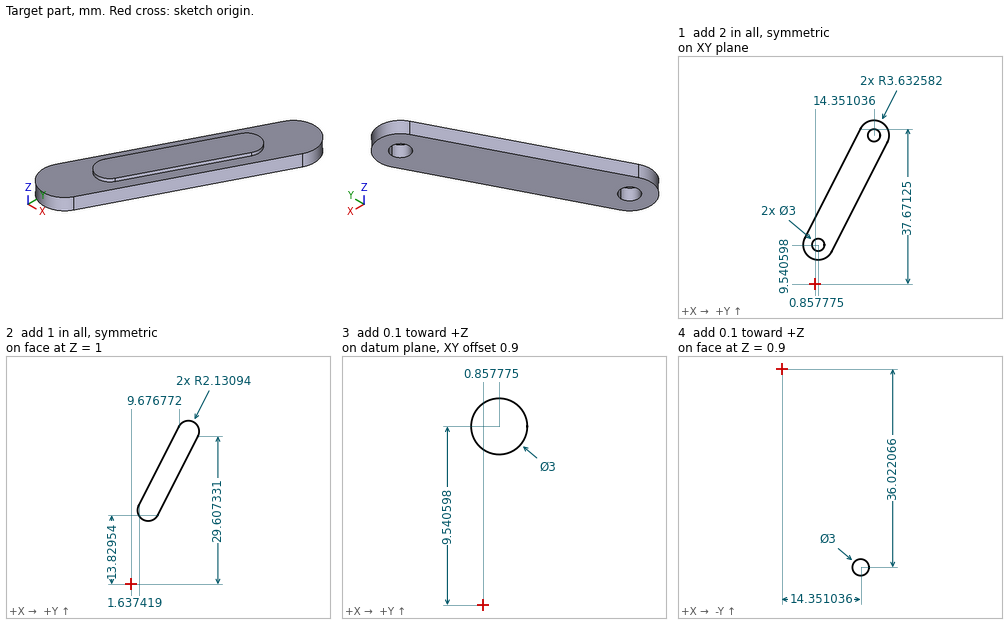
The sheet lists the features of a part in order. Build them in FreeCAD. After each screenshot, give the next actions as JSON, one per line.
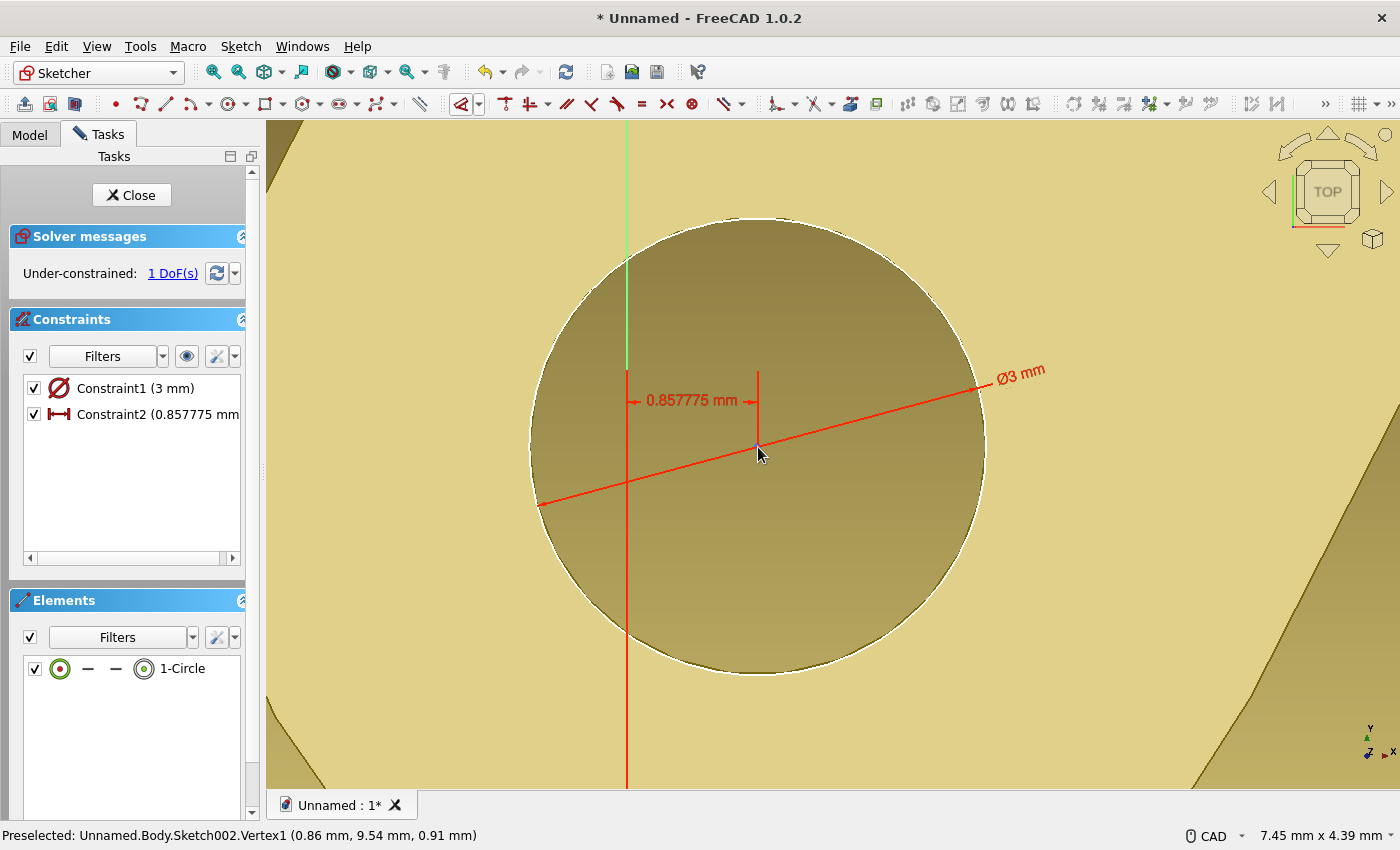
{"action": "left_click", "coordinate": [758, 447]}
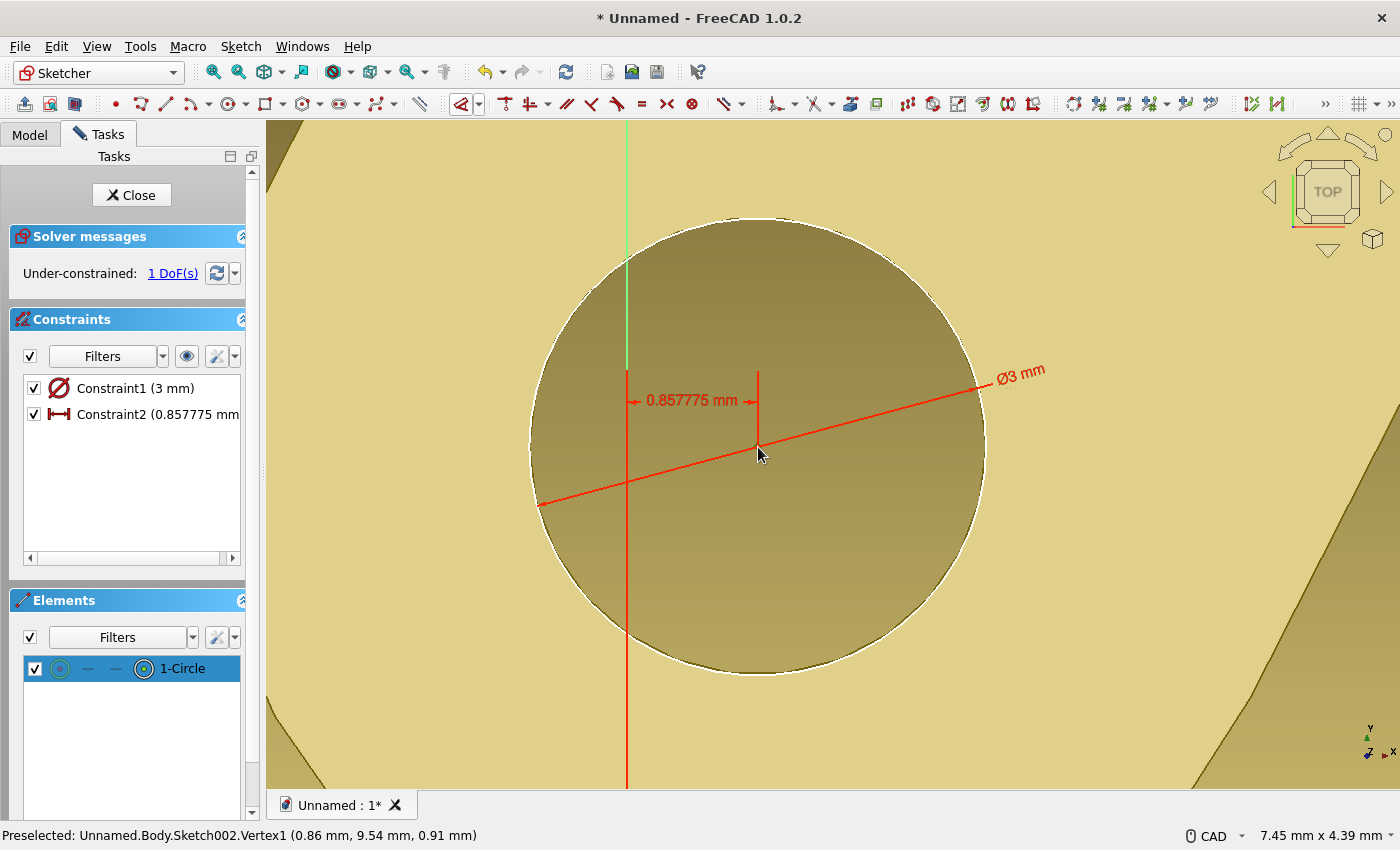
{"action": "left_click", "coordinate": [478, 104]}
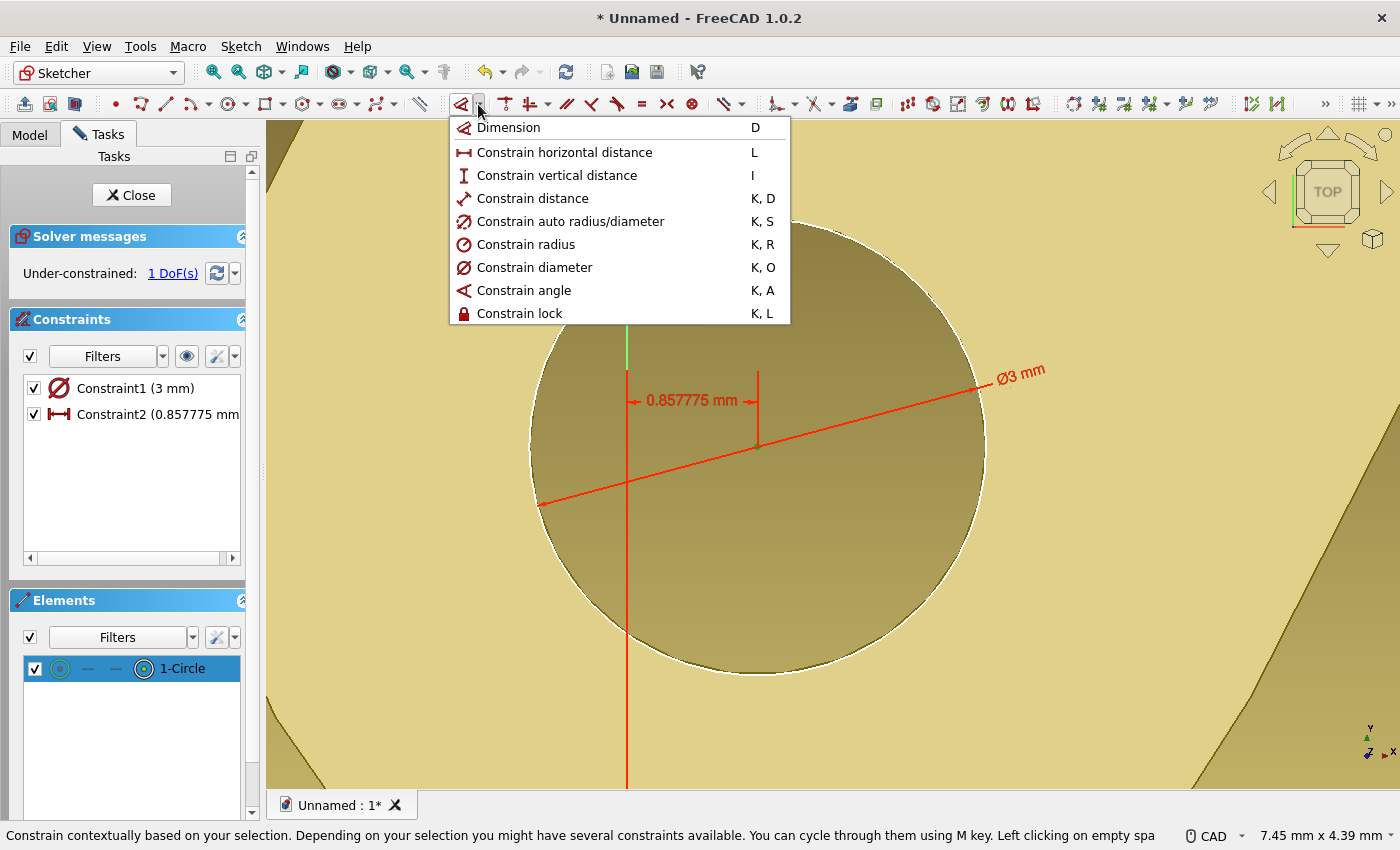
{"action": "left_click", "coordinate": [620, 176]}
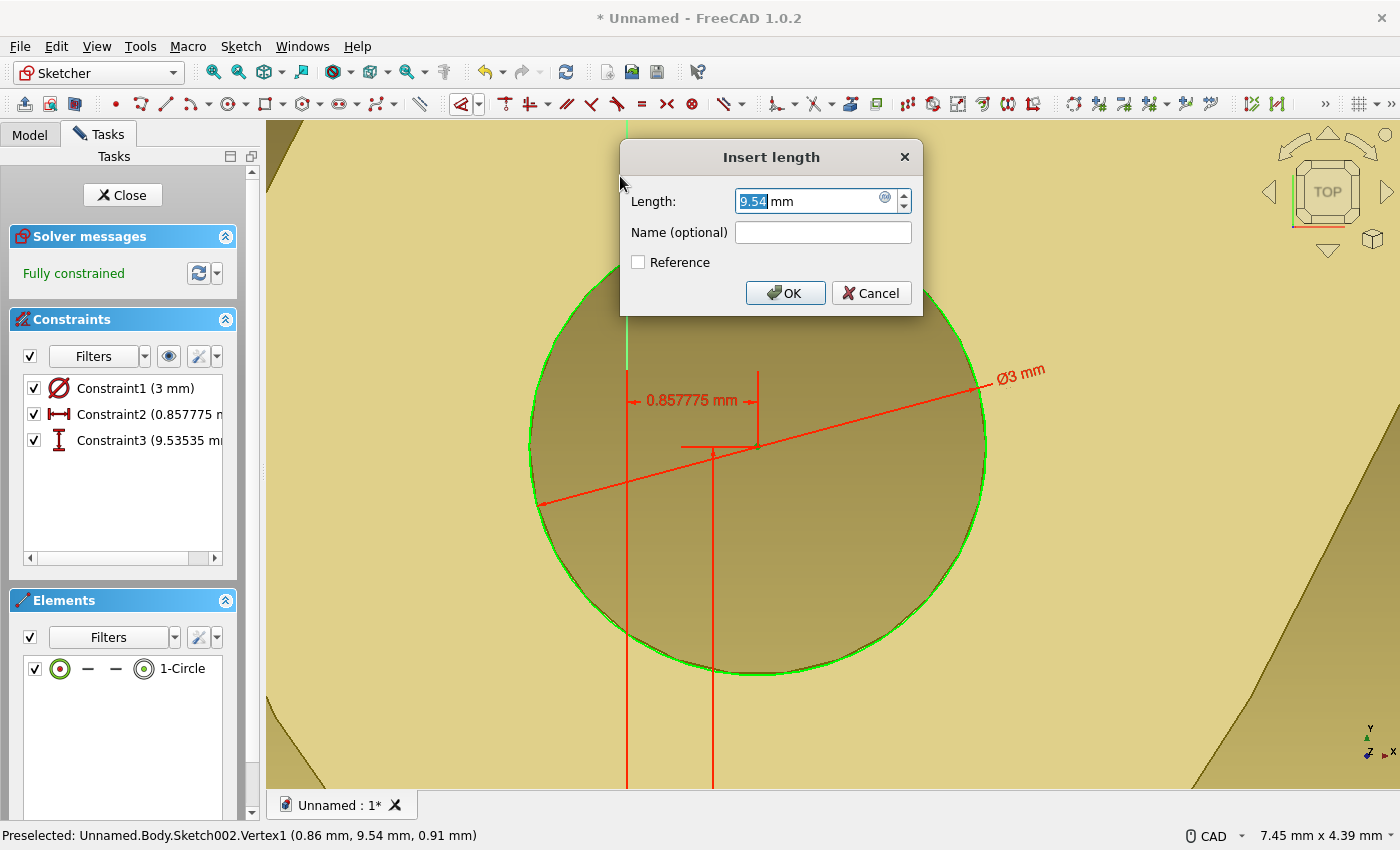
{"action": "type", "text": "9.540598"}
{"action": "key", "text": "Return"}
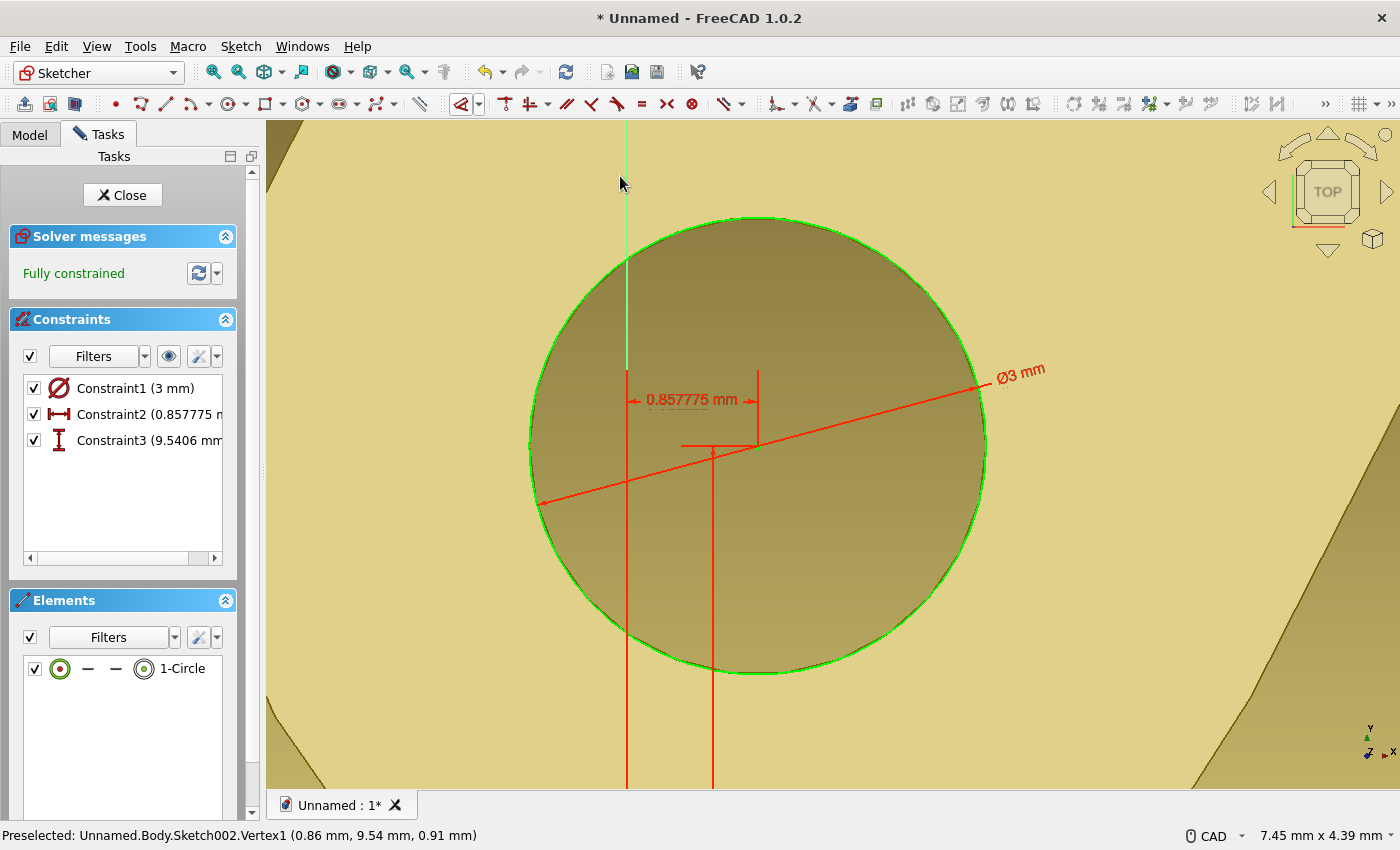
{"action": "left_click", "coordinate": [123, 195]}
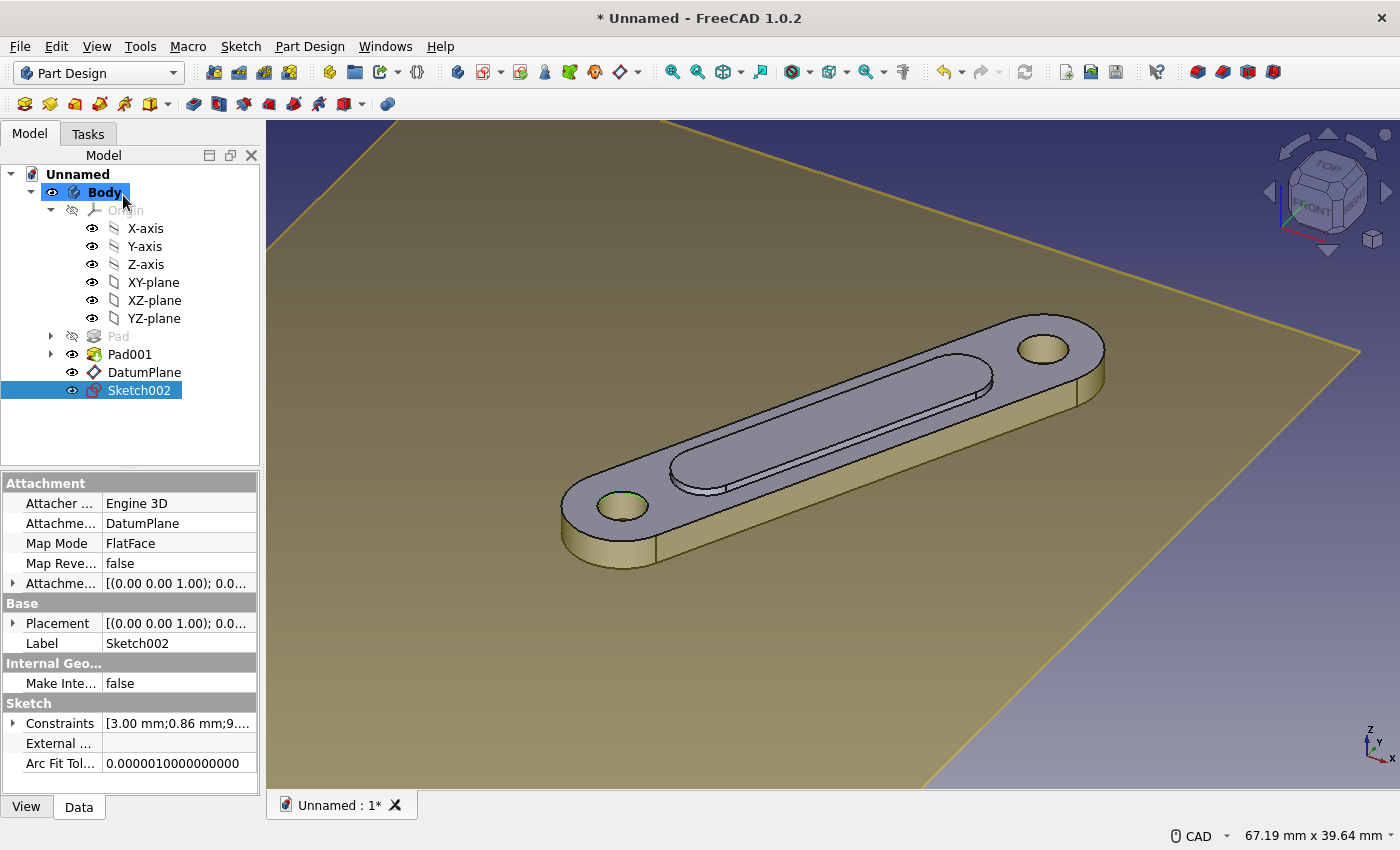
{"action": "left_click", "coordinate": [25, 104]}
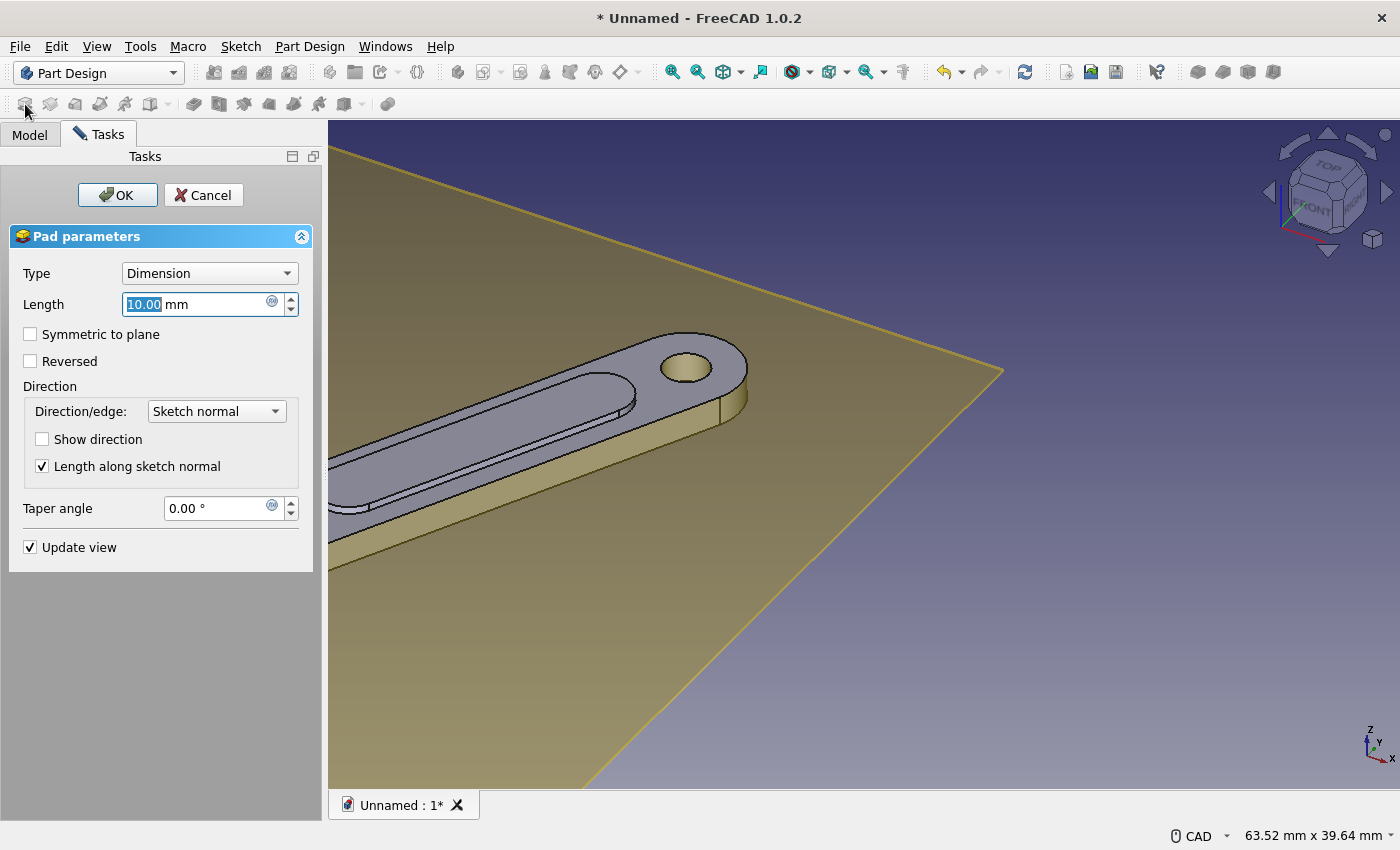
{"action": "type", "text": "0.1"}
{"action": "key", "text": "Tab"}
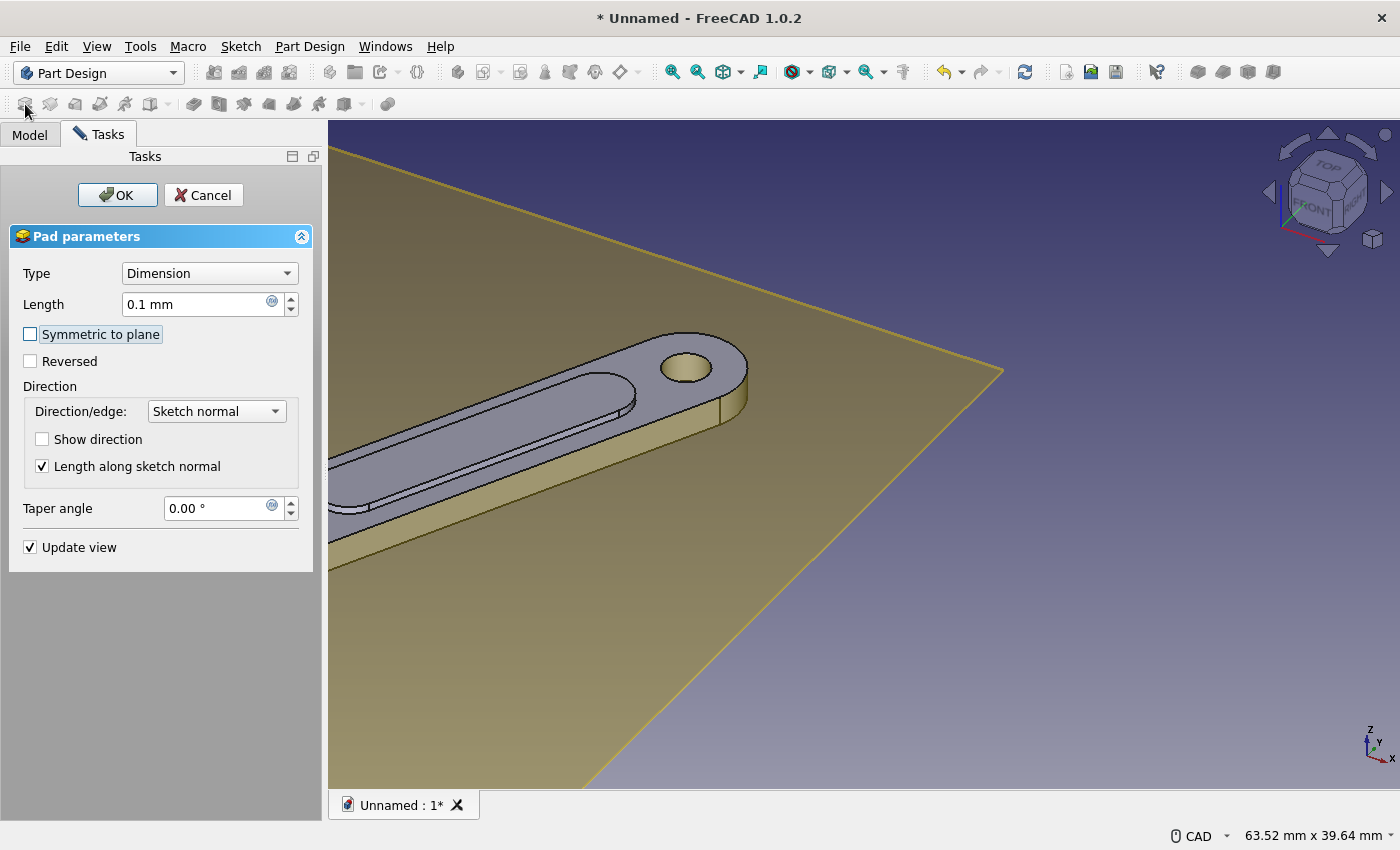
{"action": "left_click", "coordinate": [118, 195]}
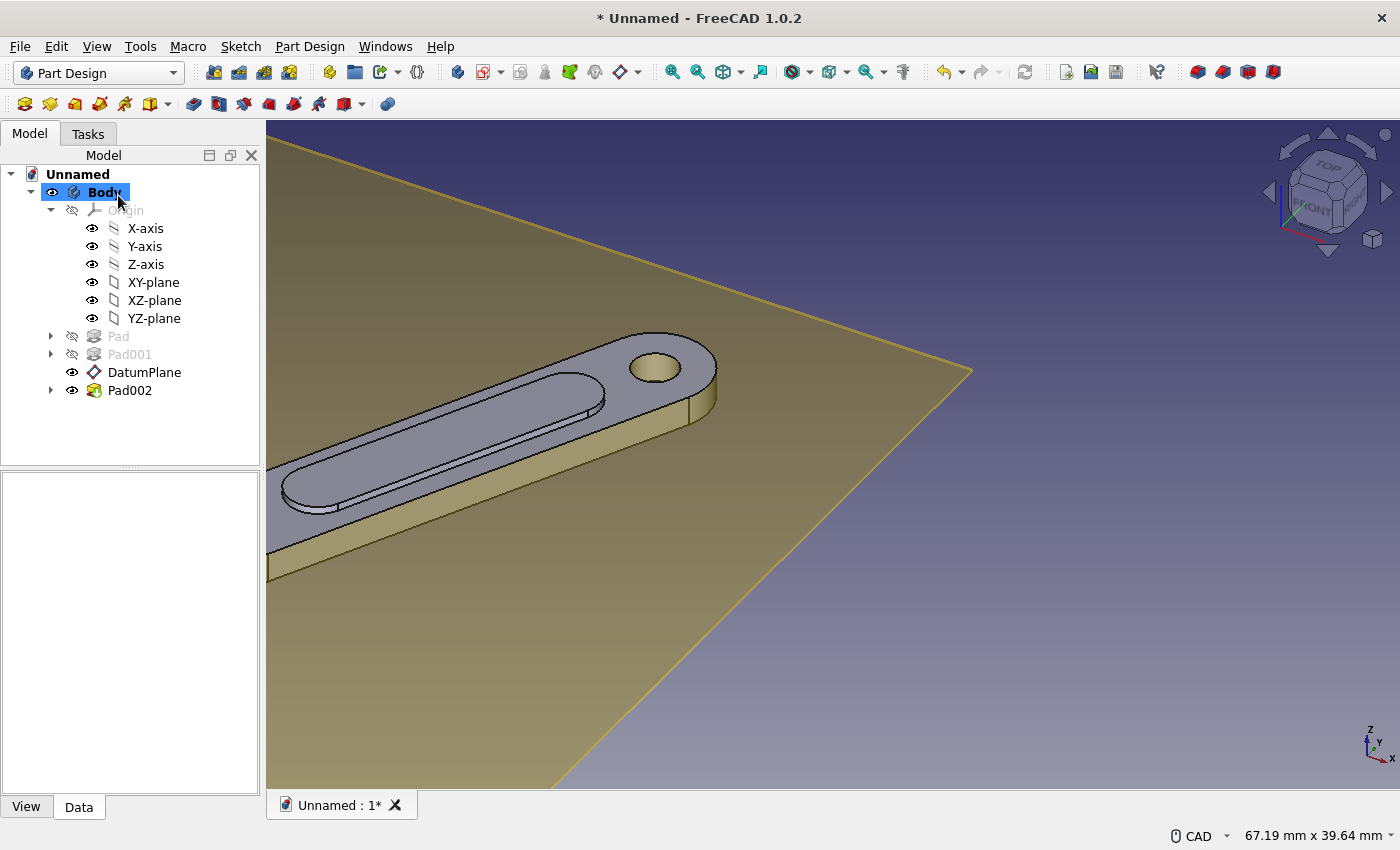
{"action": "left_click", "coordinate": [117, 372]}
{"action": "key", "text": "space"}